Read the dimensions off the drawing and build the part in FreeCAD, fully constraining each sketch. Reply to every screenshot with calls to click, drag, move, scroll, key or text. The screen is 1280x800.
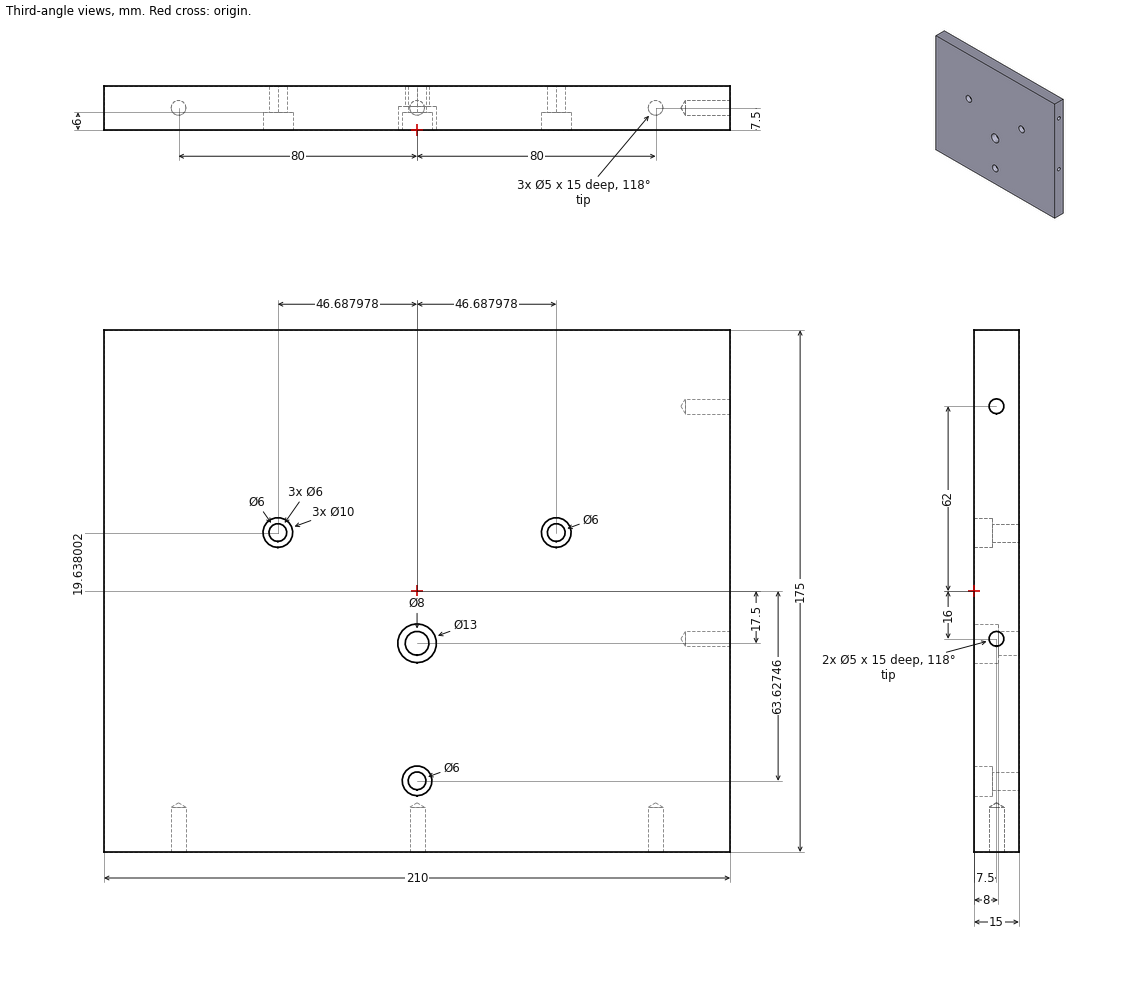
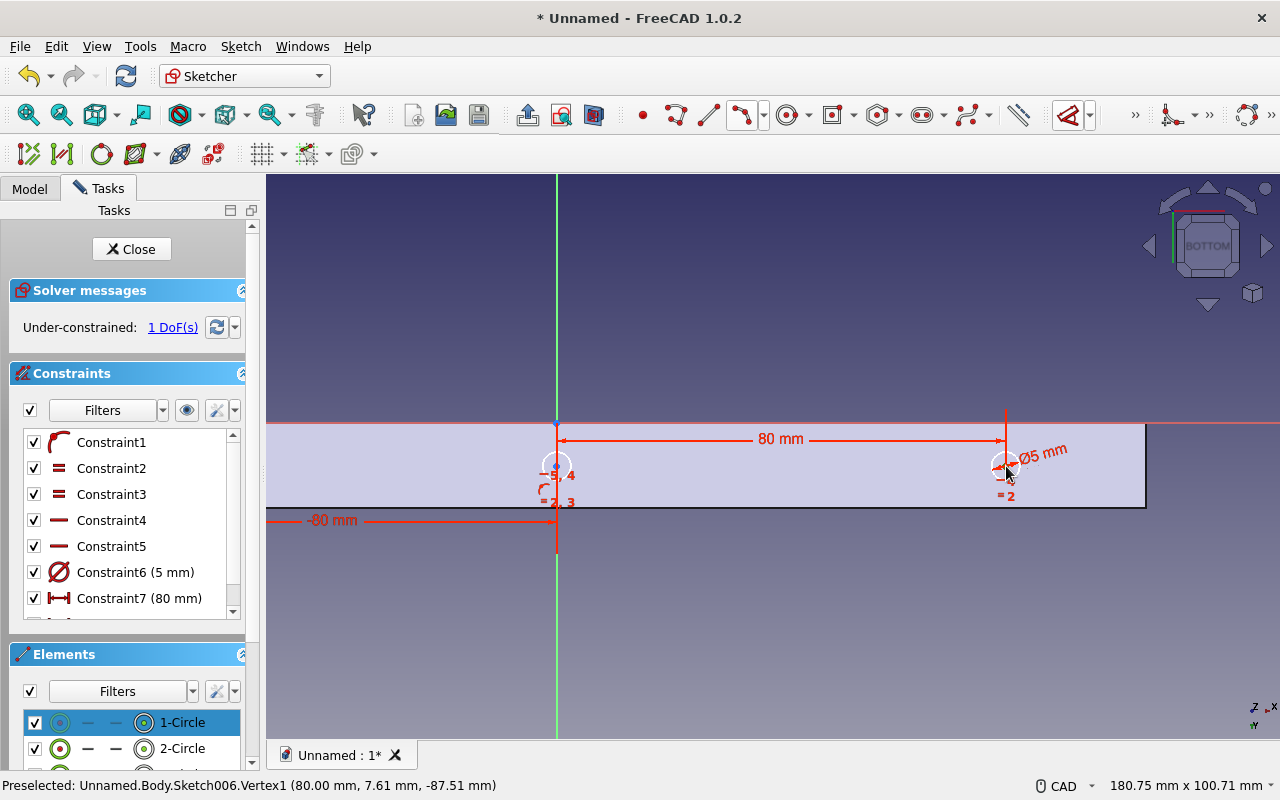
click(1090, 116)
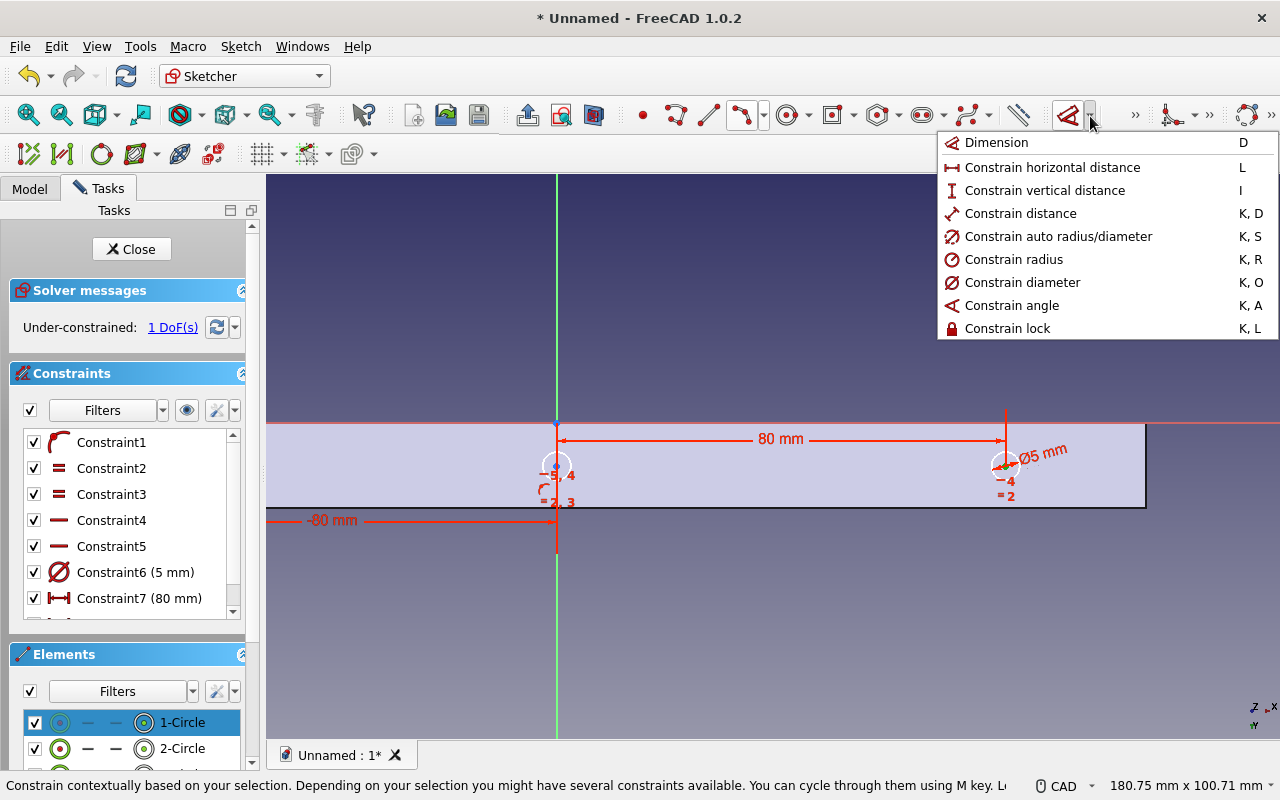
click(1108, 190)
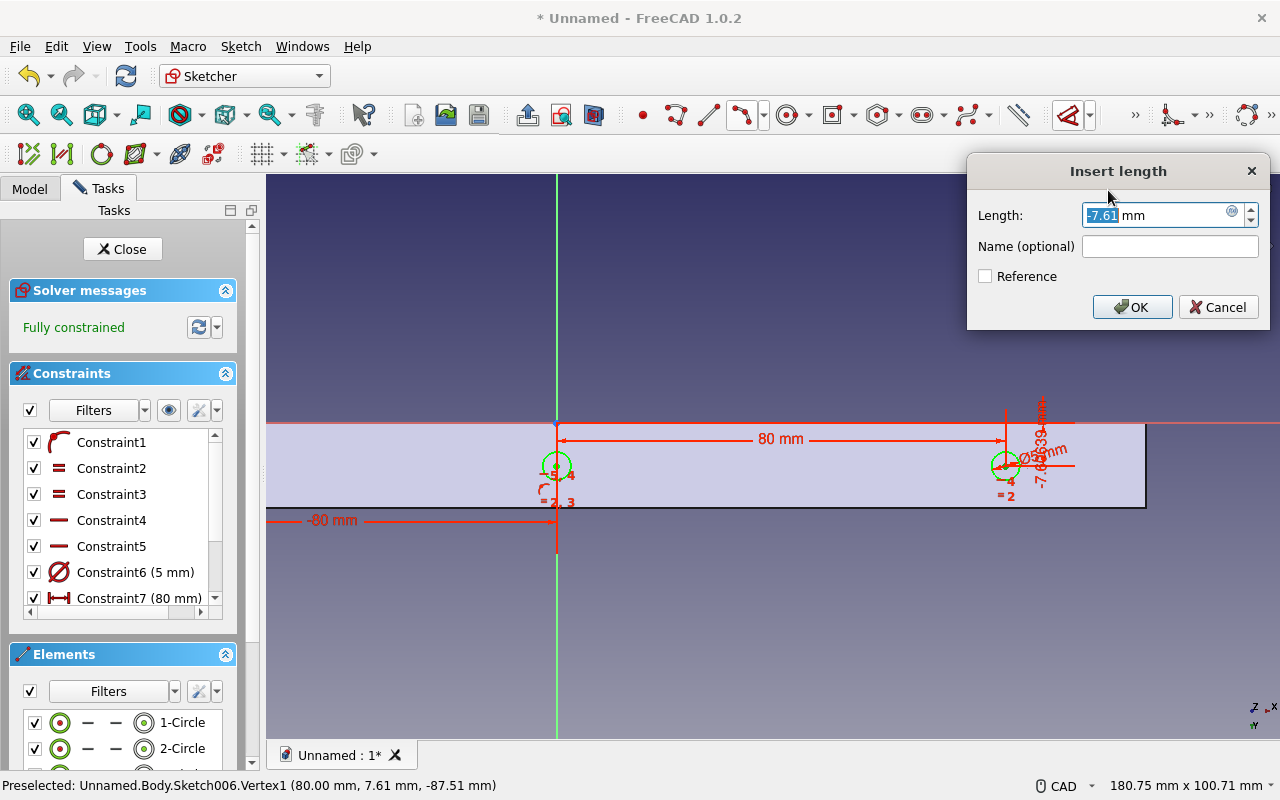
text(-7.5)
key(Return)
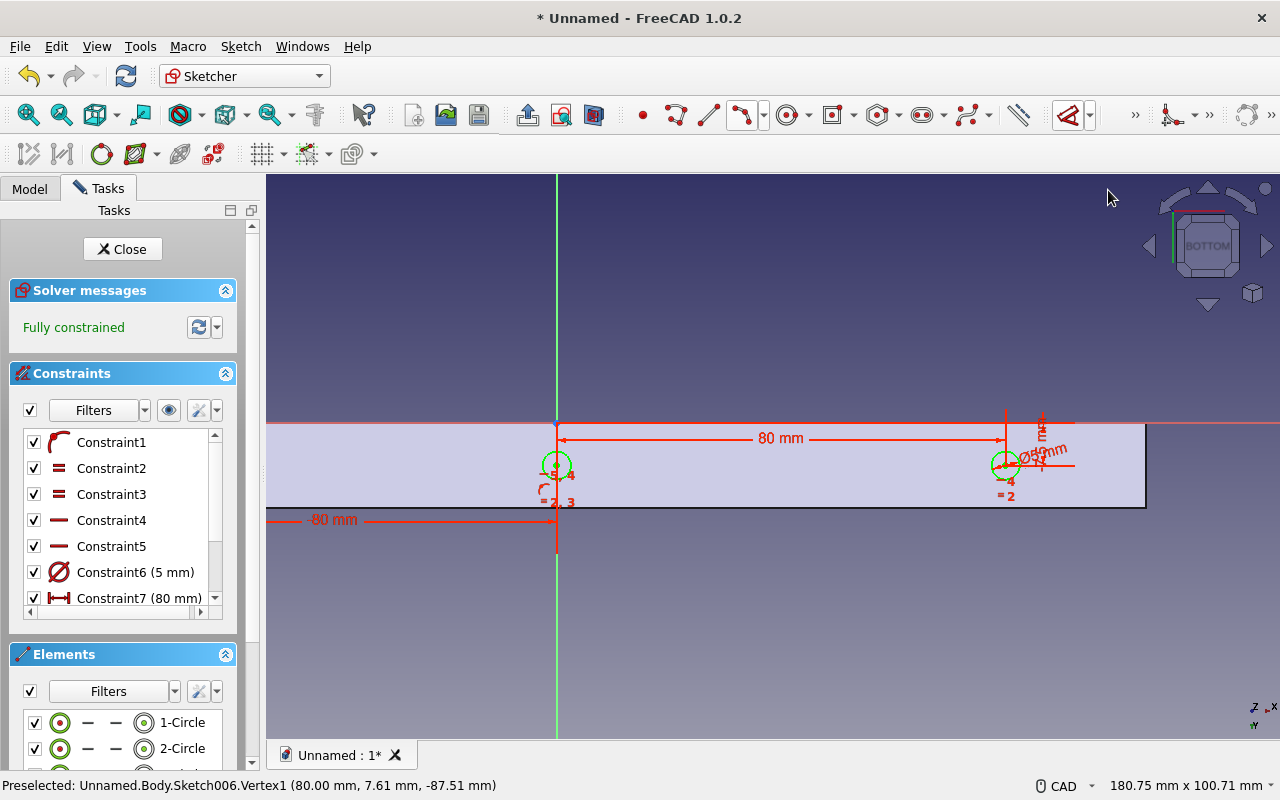
click(123, 249)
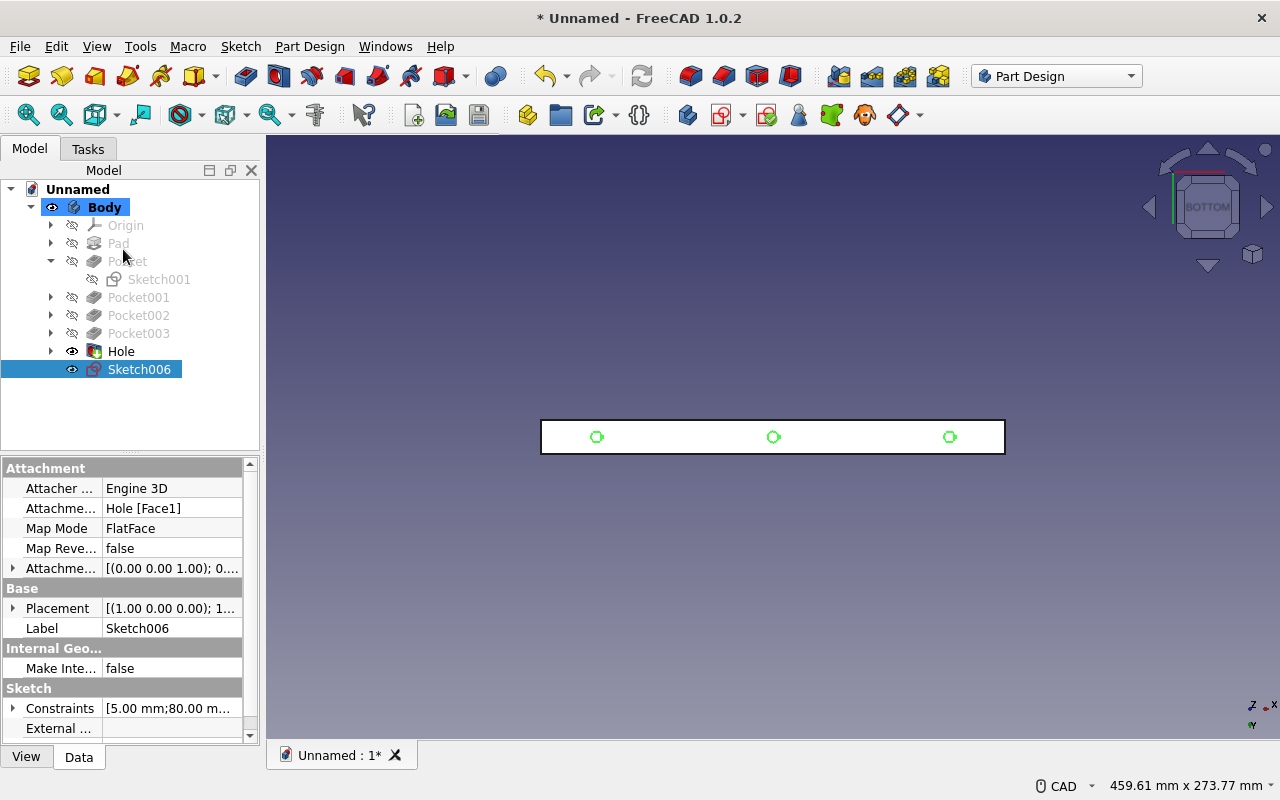
click(279, 76)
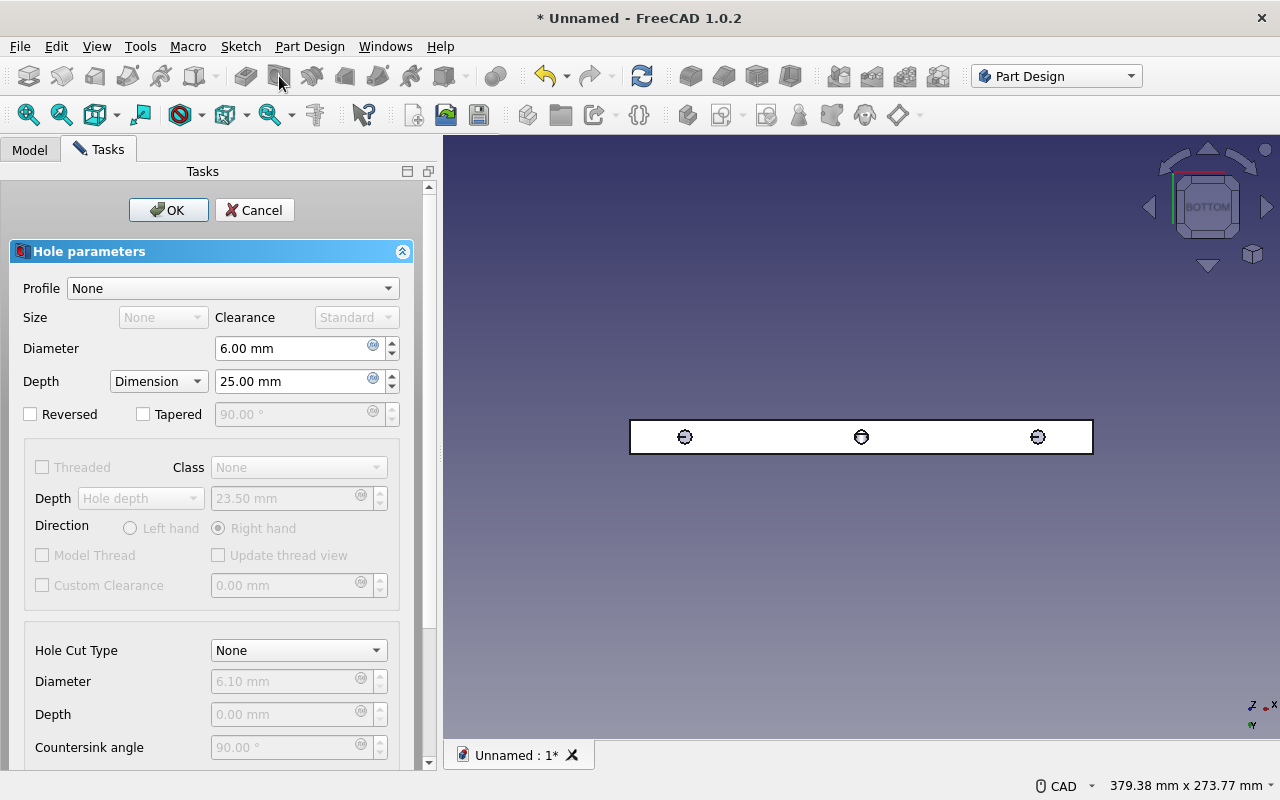
triple_click(300, 348)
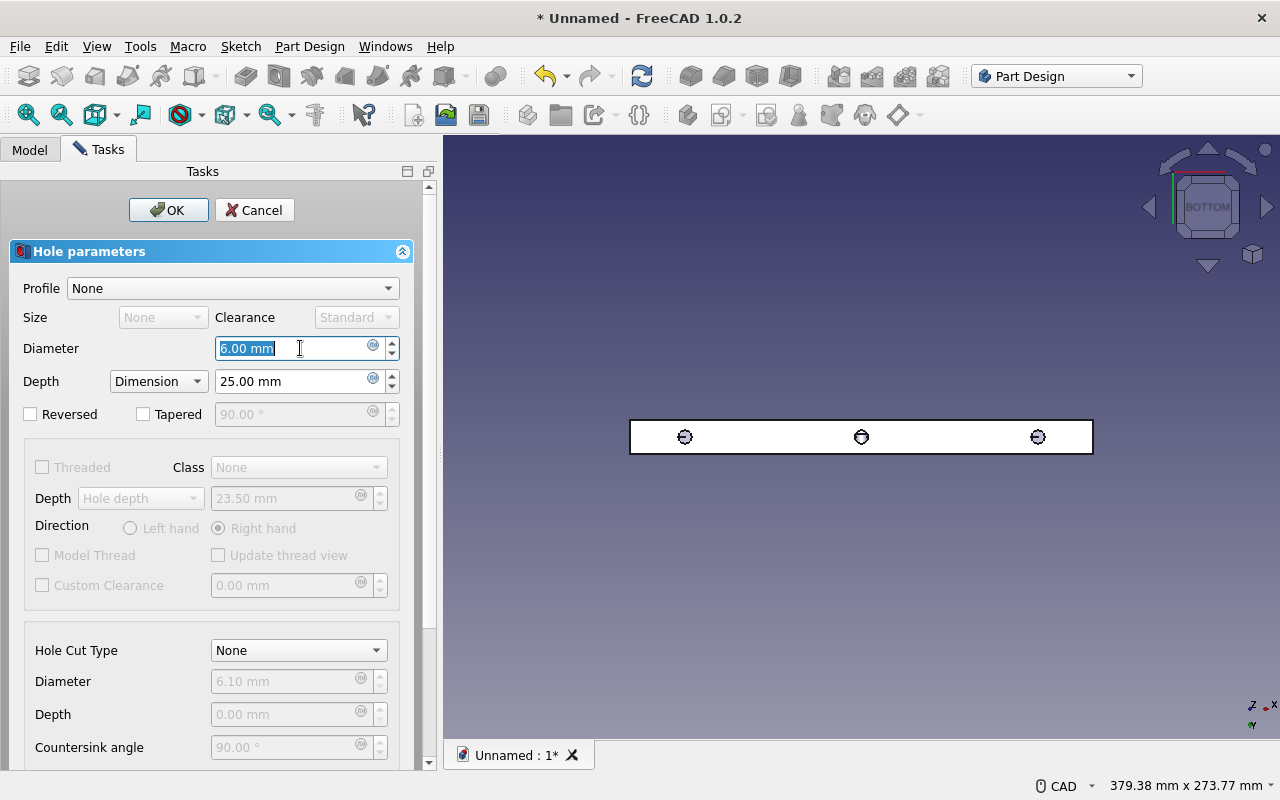
text(5)
key(Tab)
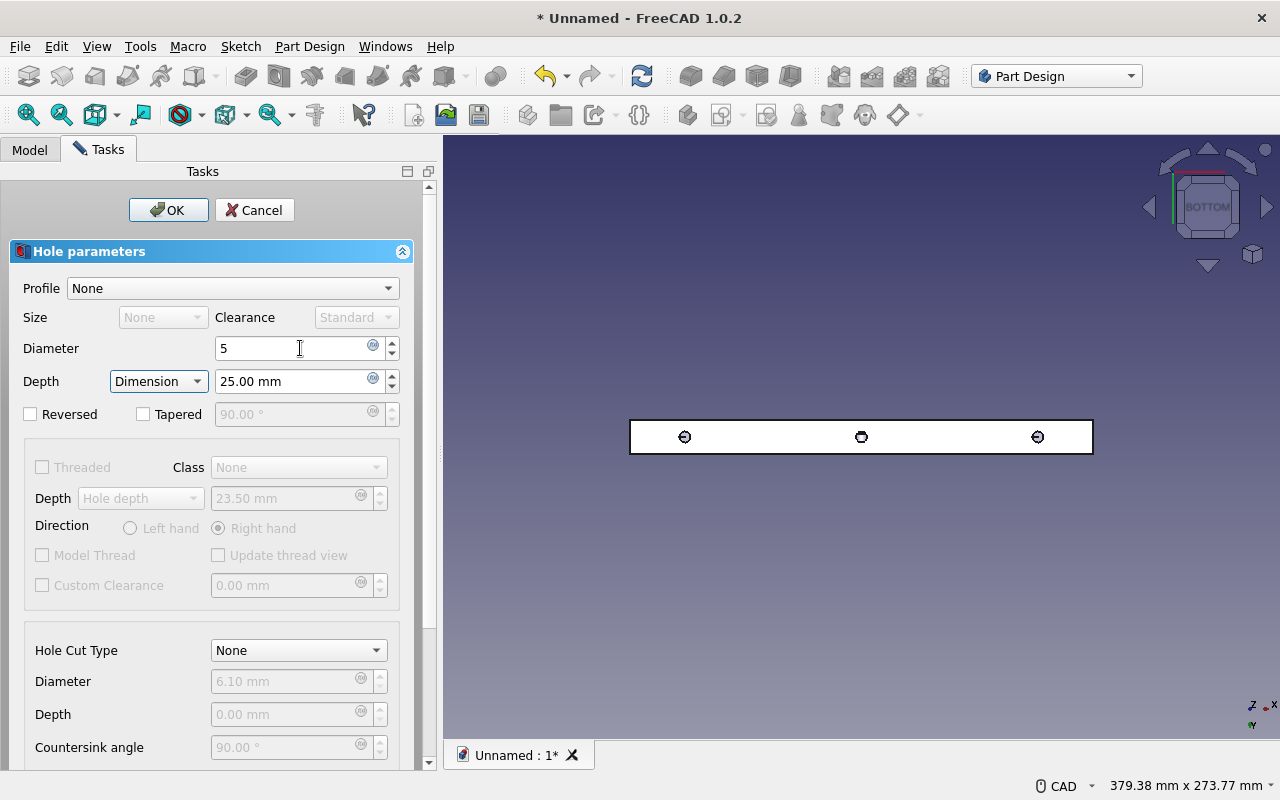
triple_click(300, 382)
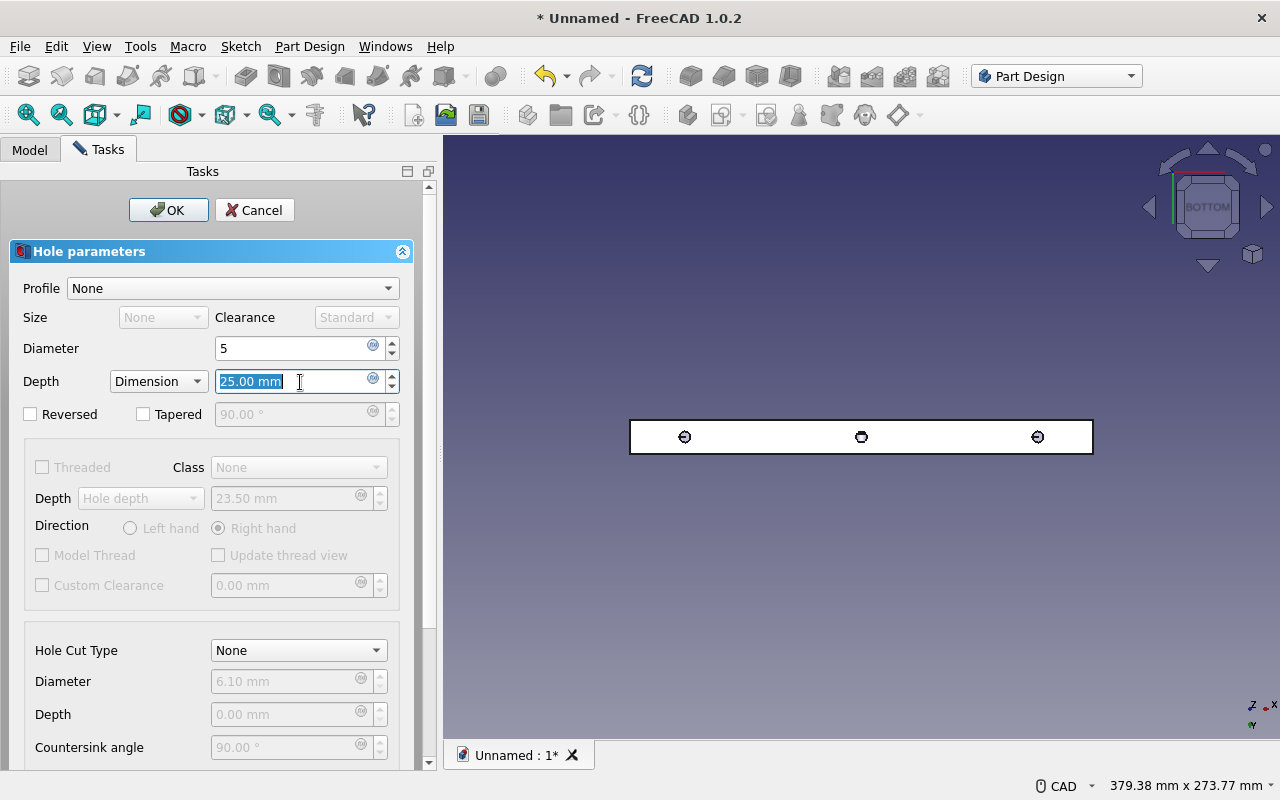
text(15)
key(Tab)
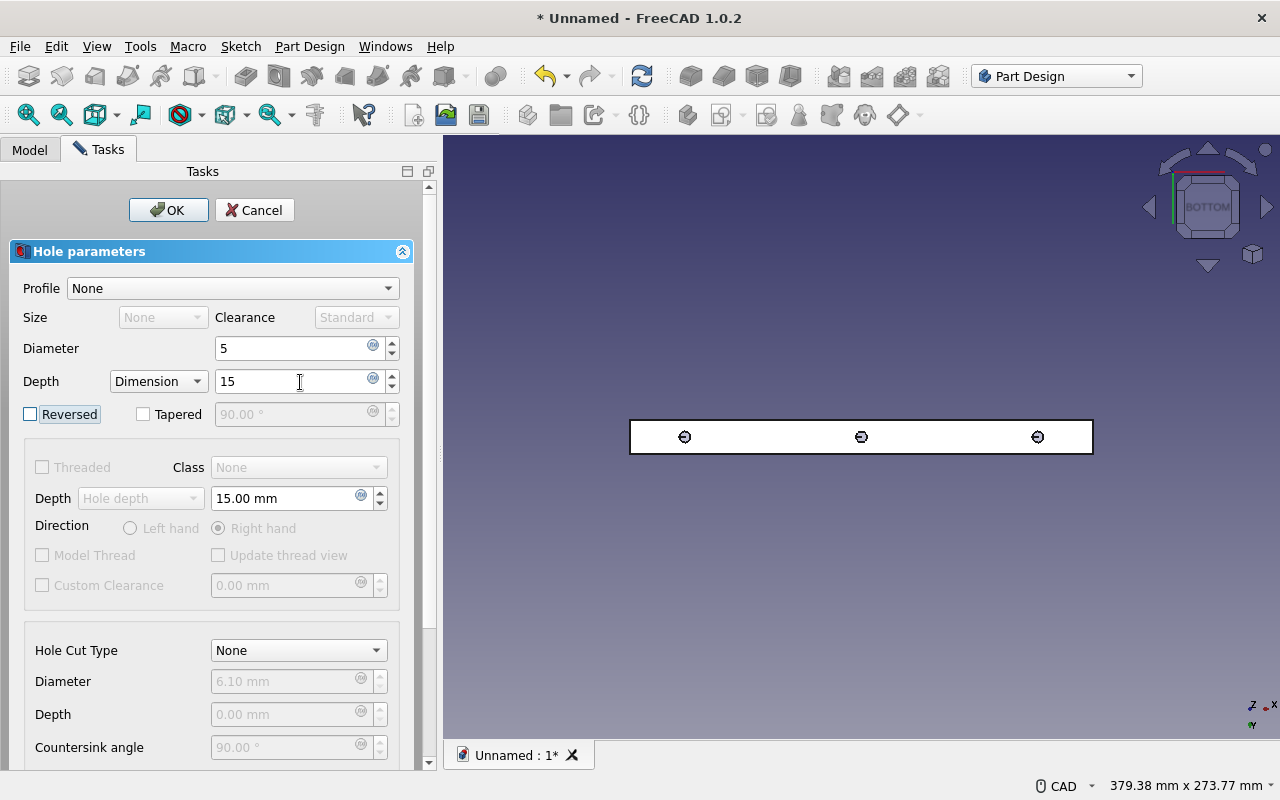
click(169, 210)